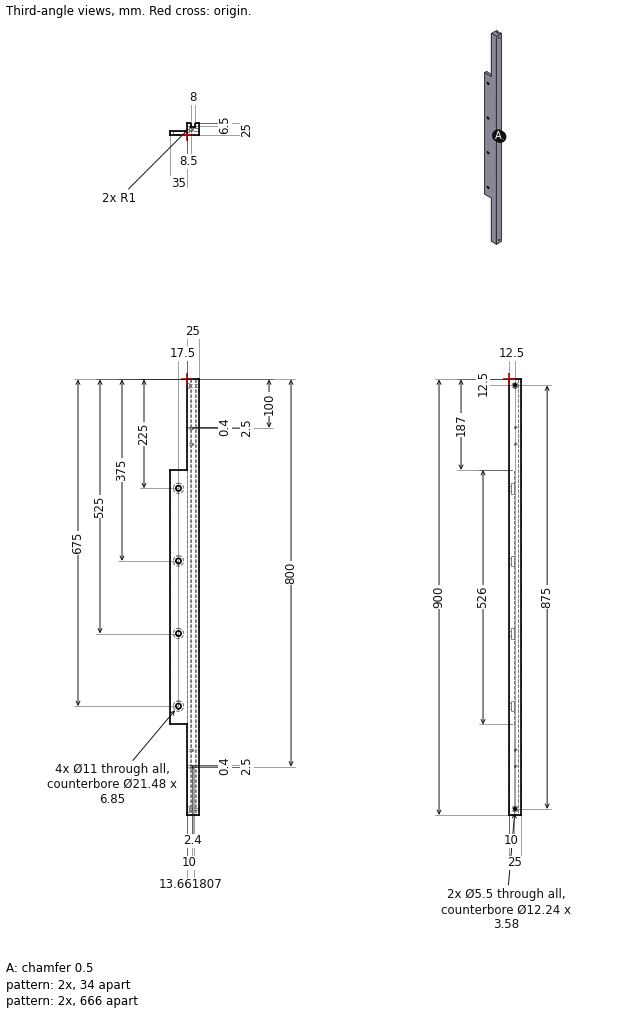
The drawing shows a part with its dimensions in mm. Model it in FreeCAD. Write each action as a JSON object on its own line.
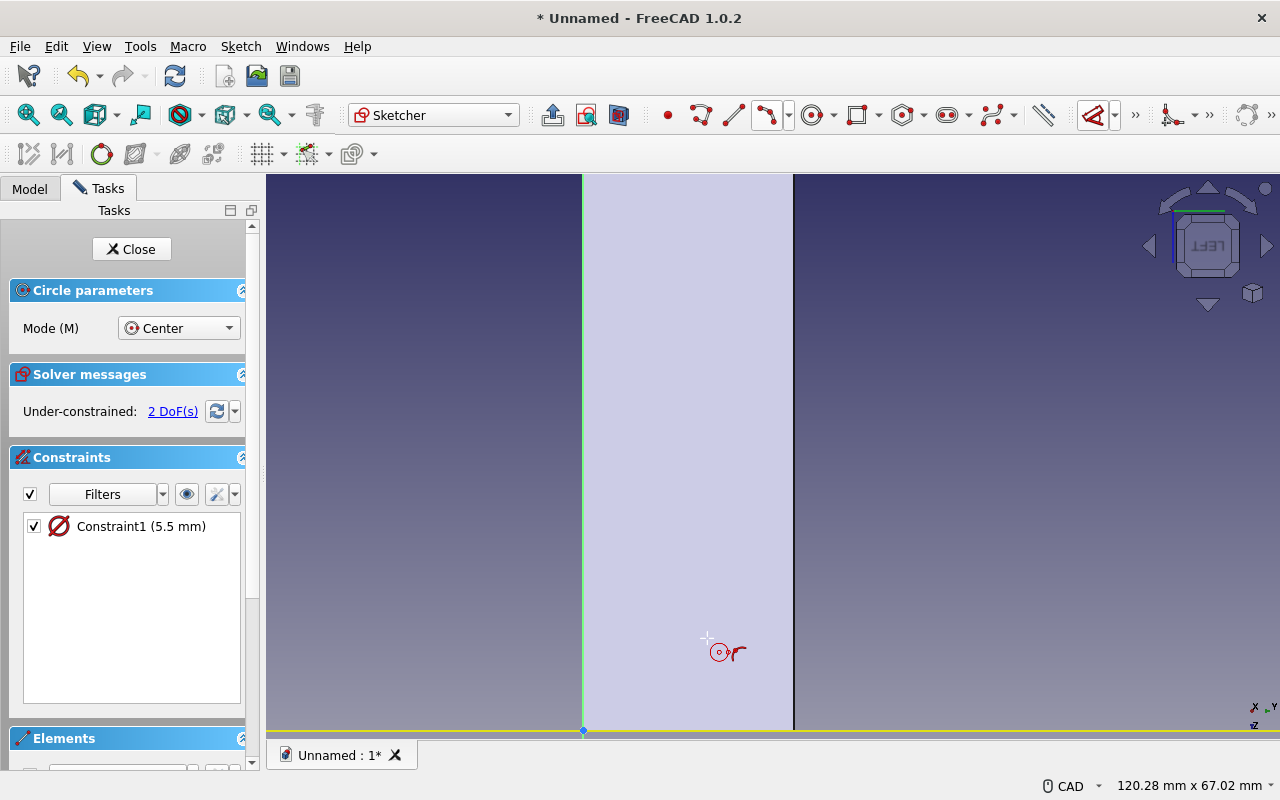
{"action": "scroll", "coordinate": [707, 639], "scroll_direction": "down", "scroll_amount": 15}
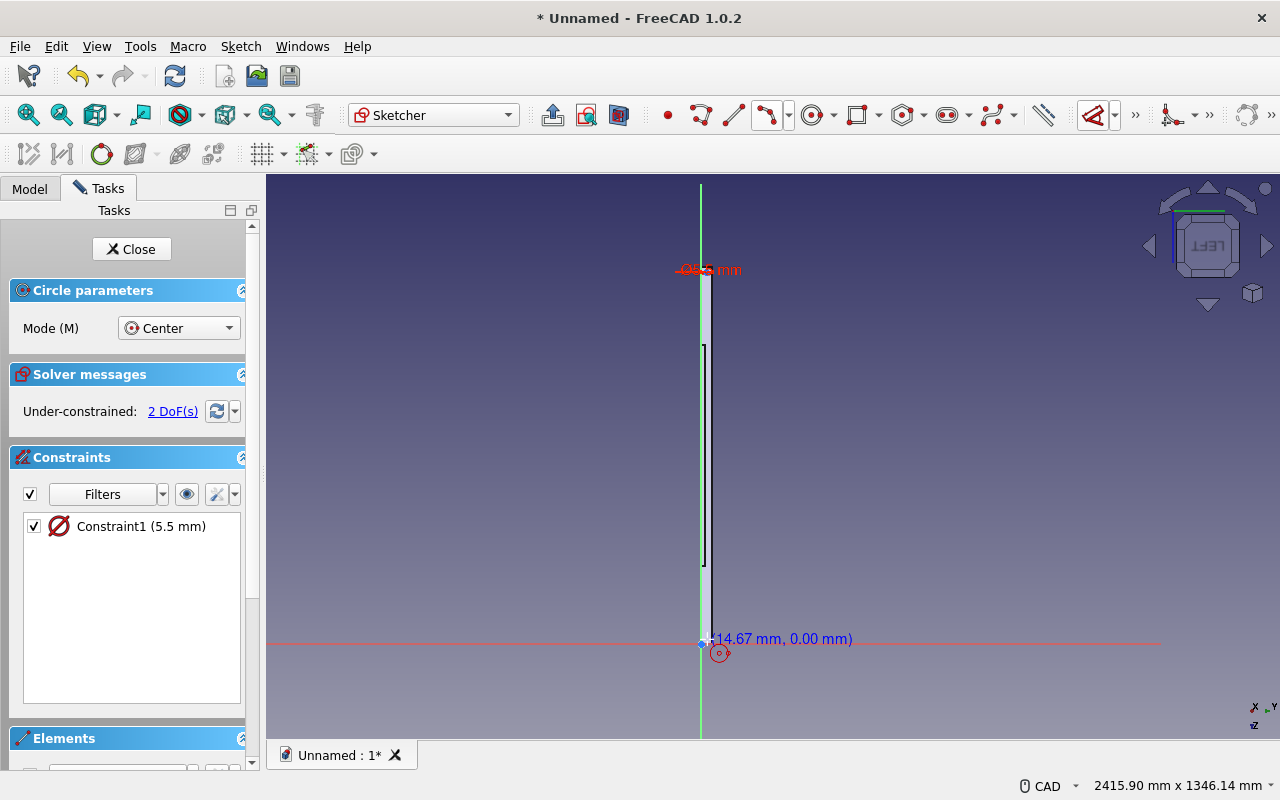
{"action": "scroll", "coordinate": [707, 639], "scroll_direction": "up", "scroll_amount": 6}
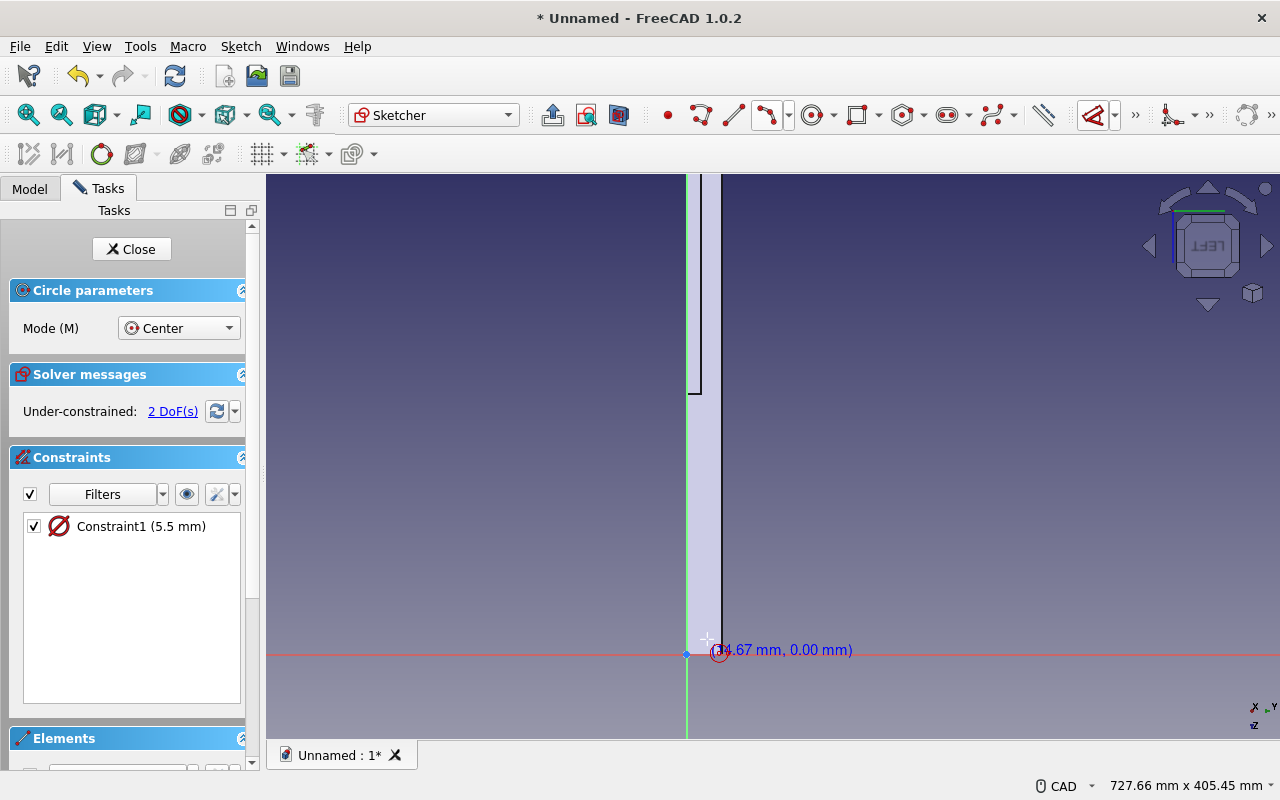
{"action": "left_click", "coordinate": [704, 637]}
{"action": "mouse_move", "coordinate": [707, 635]}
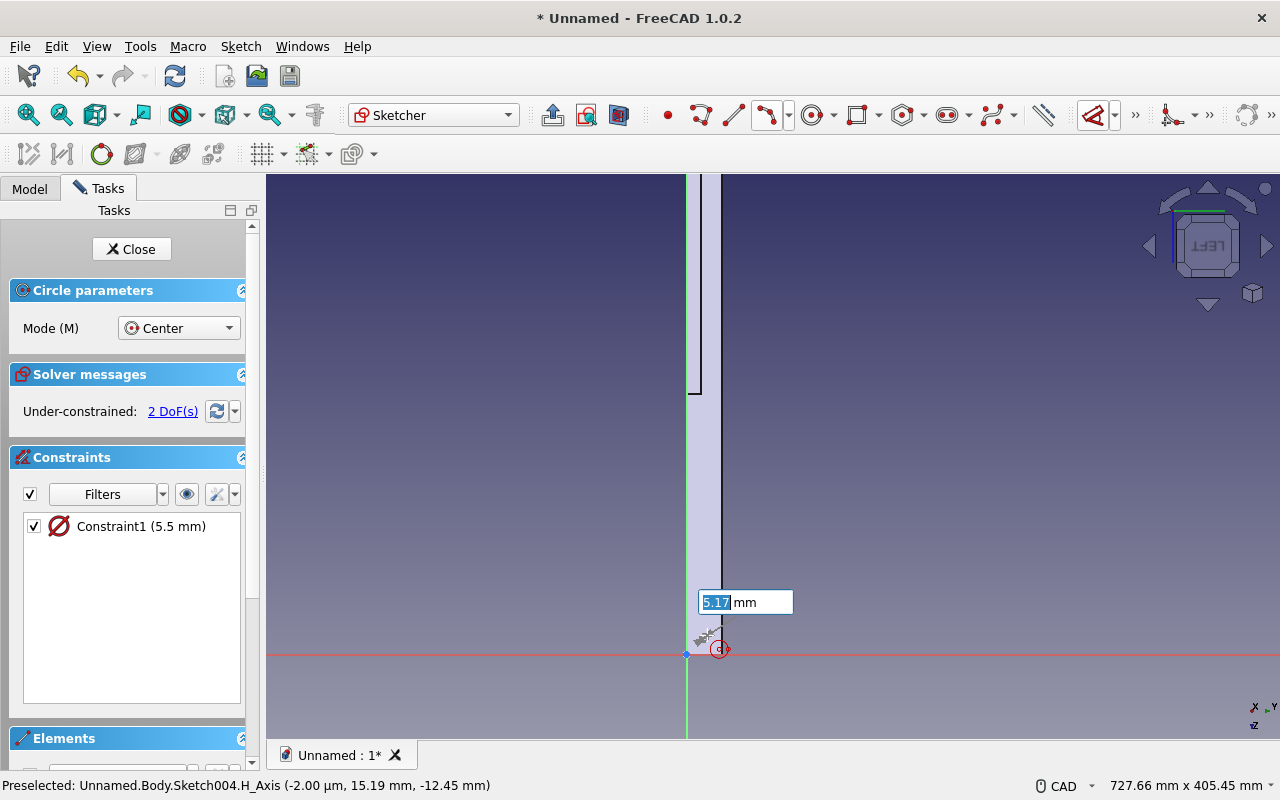
{"action": "type", "text": "5.5"}
{"action": "key", "text": "Return"}
{"action": "key", "text": "Escape"}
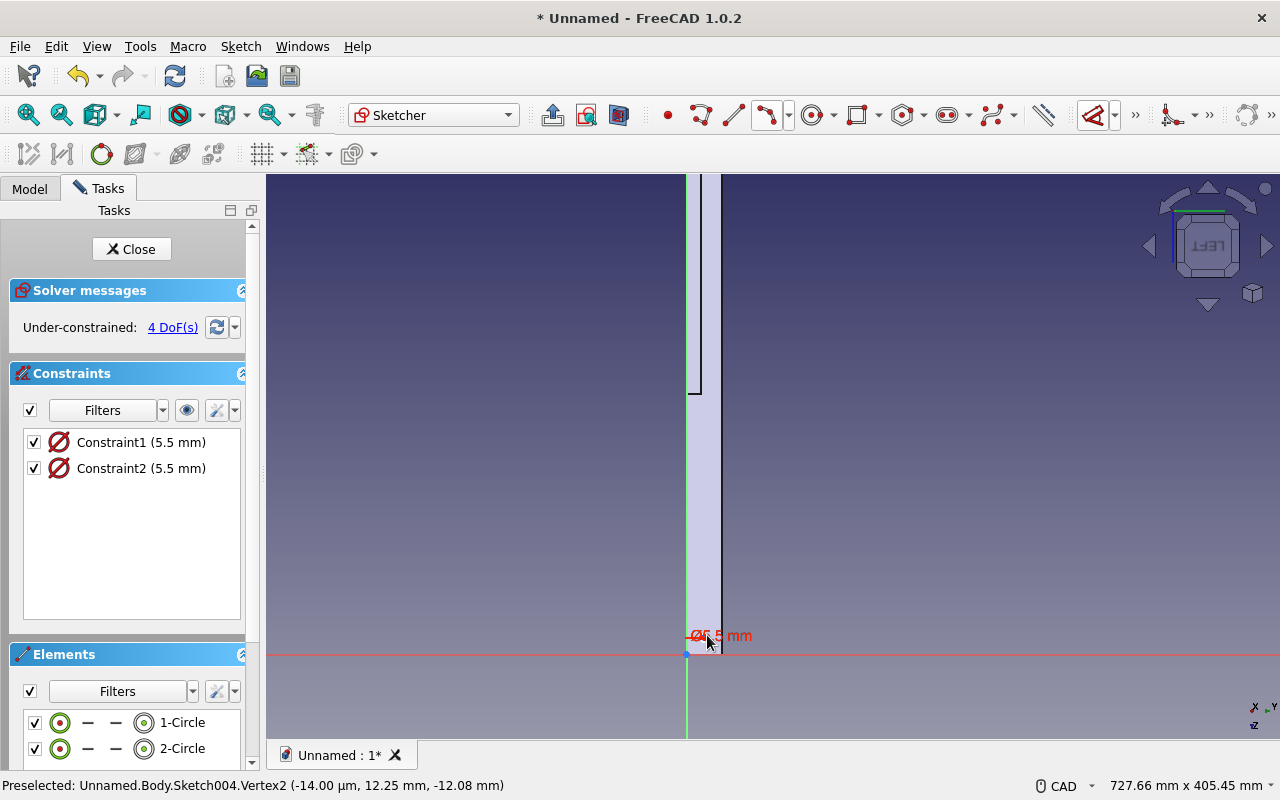
{"action": "scroll", "coordinate": [707, 638], "scroll_direction": "down", "scroll_amount": 6}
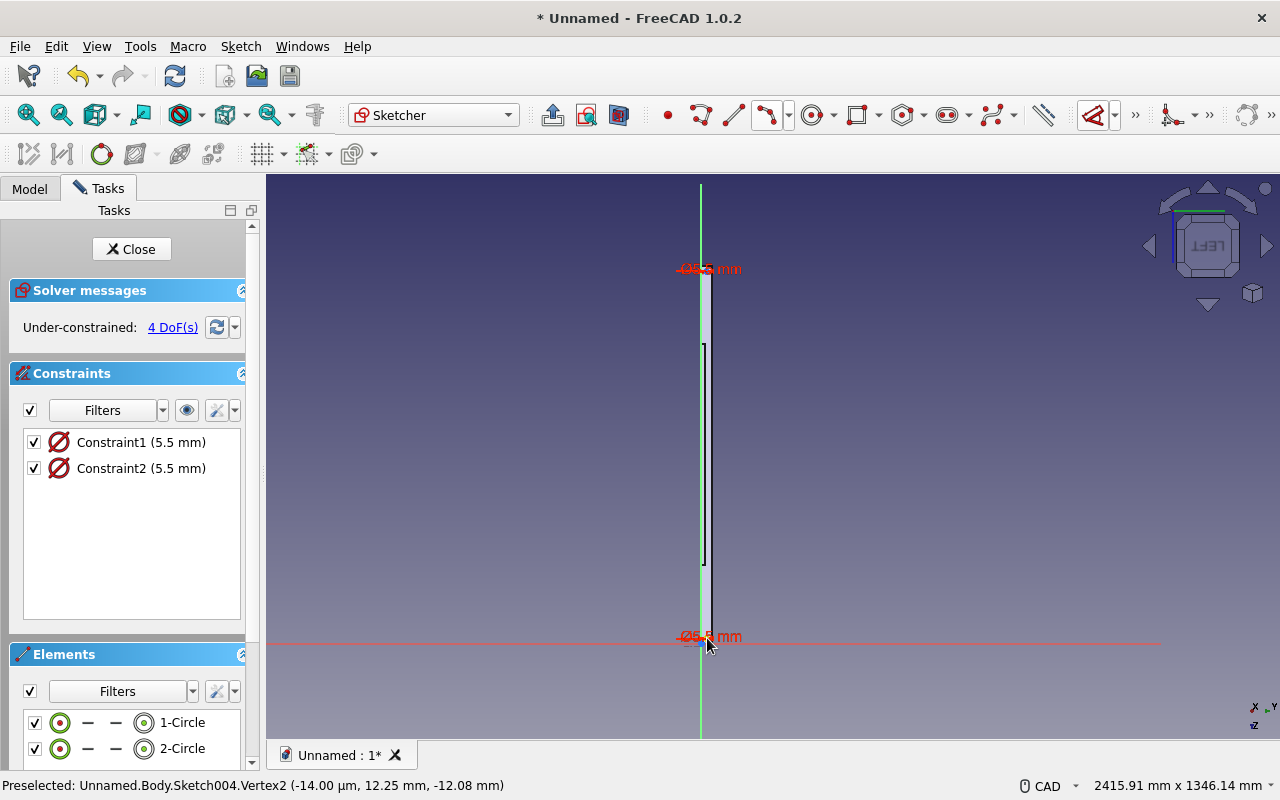
{"action": "left_click", "coordinate": [706, 271]}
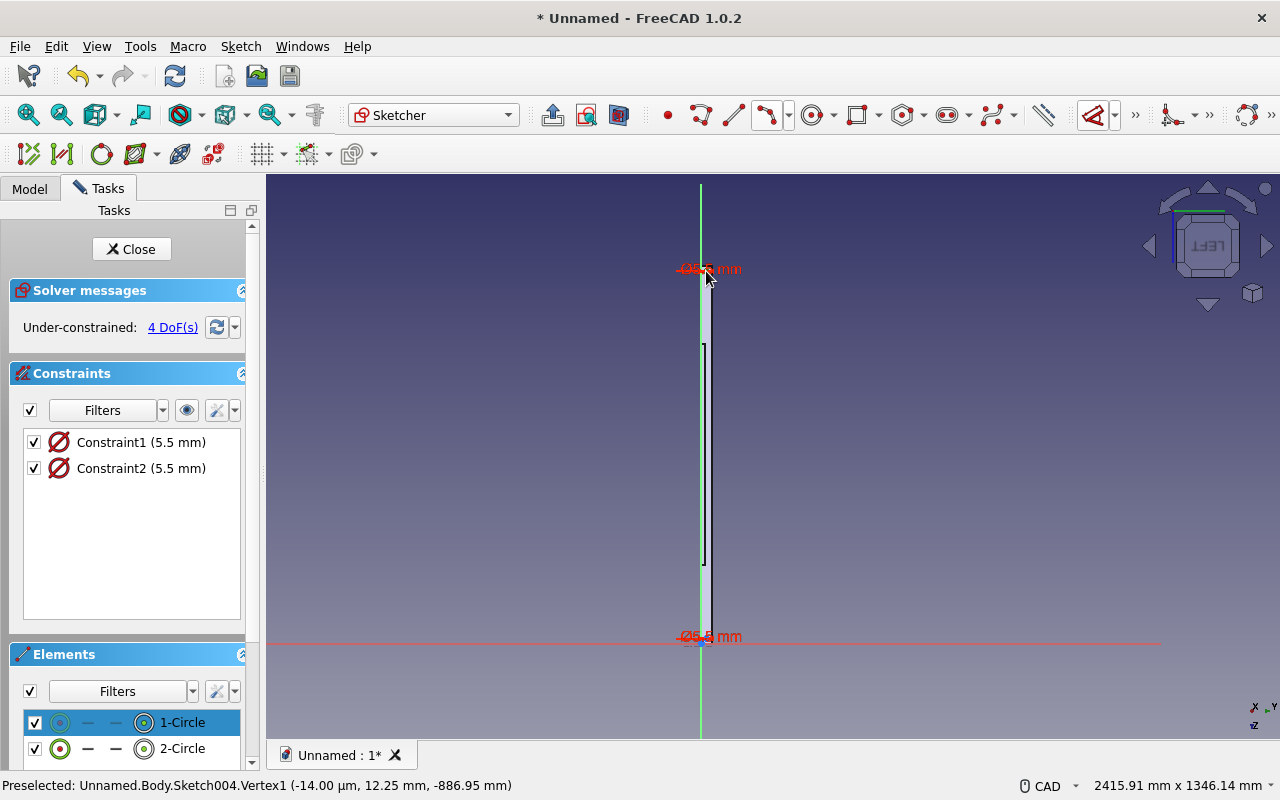
{"action": "scroll", "coordinate": [706, 639], "scroll_direction": "up", "scroll_amount": 3}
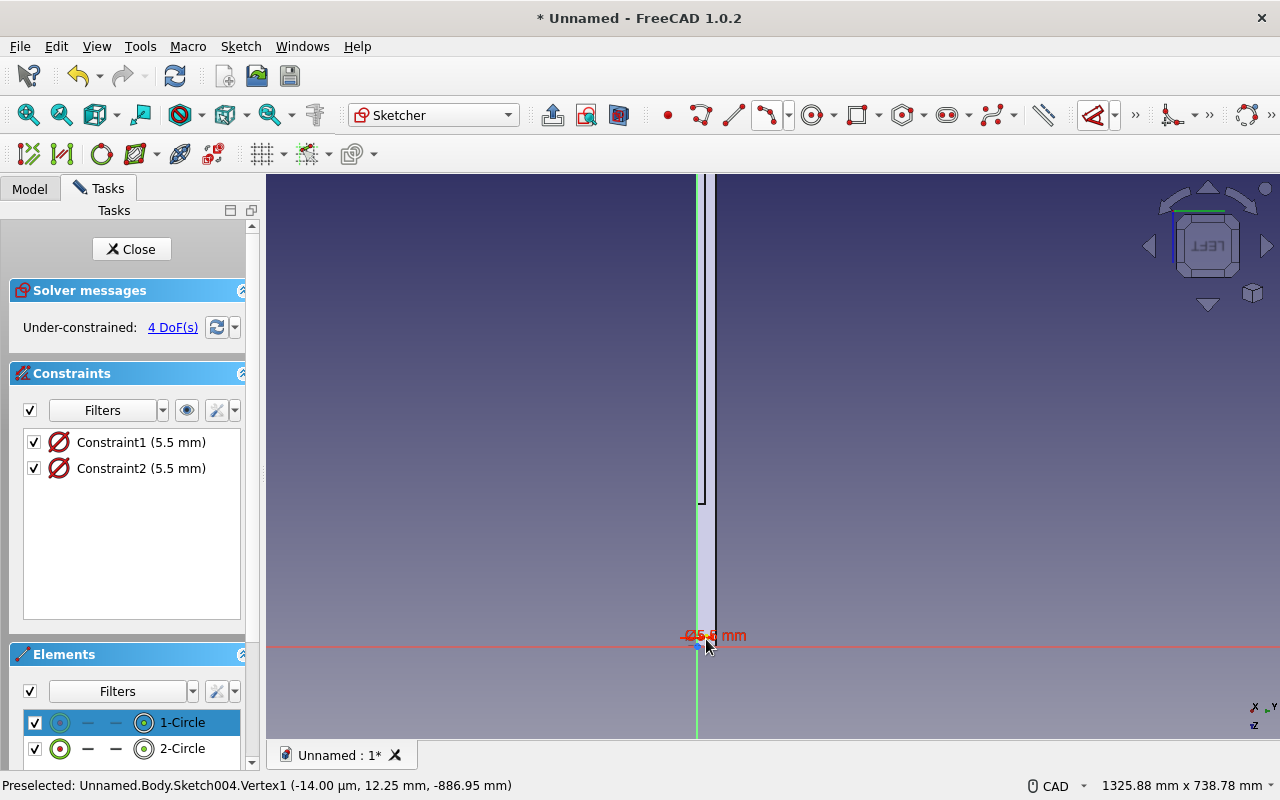
{"action": "left_click", "coordinate": [706, 638]}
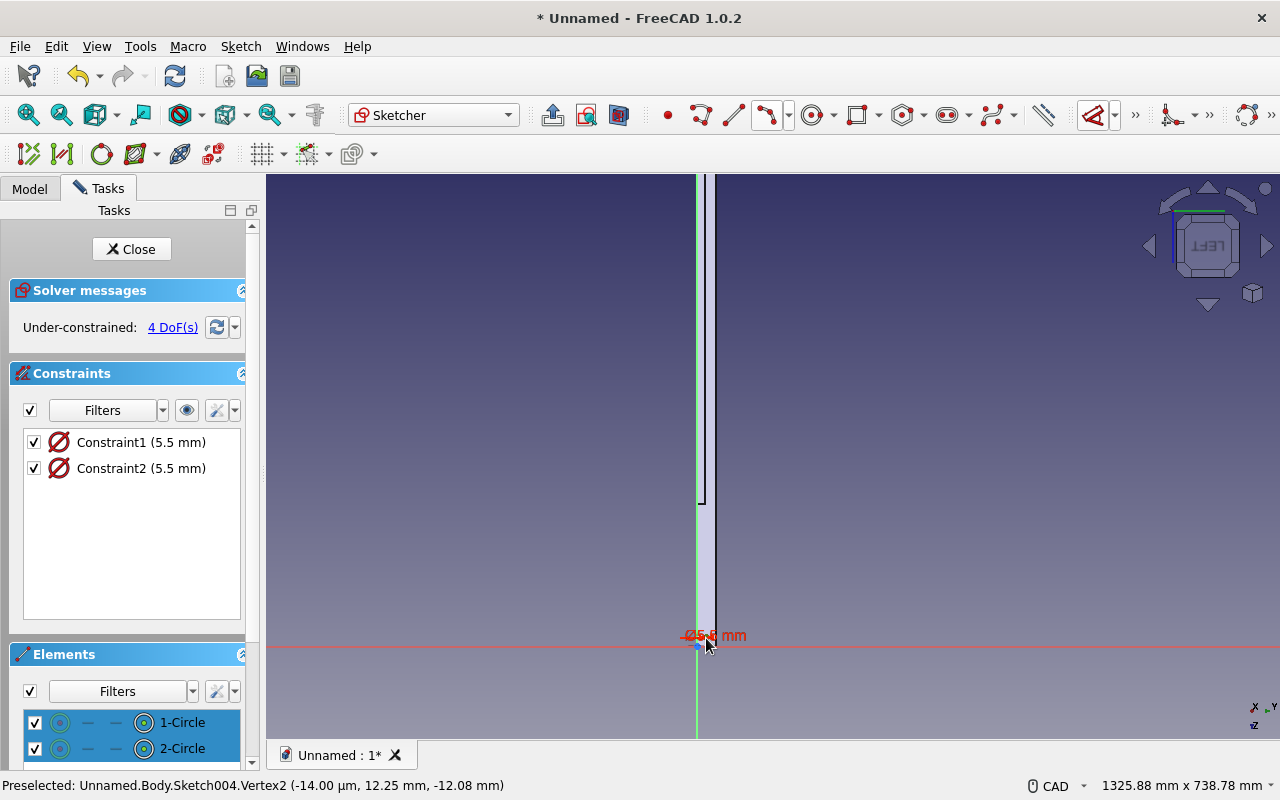
{"action": "key", "text": "v"}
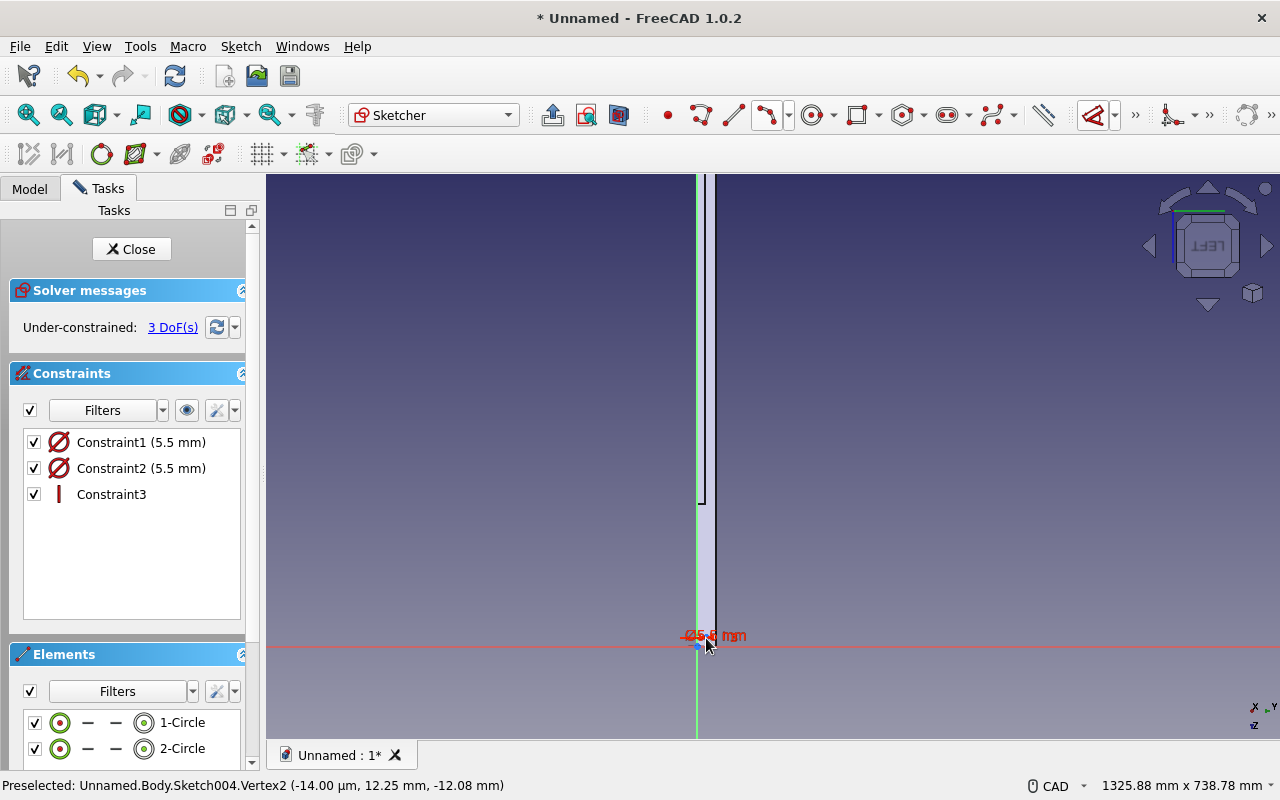
{"action": "scroll", "coordinate": [707, 639], "scroll_direction": "down", "scroll_amount": 3}